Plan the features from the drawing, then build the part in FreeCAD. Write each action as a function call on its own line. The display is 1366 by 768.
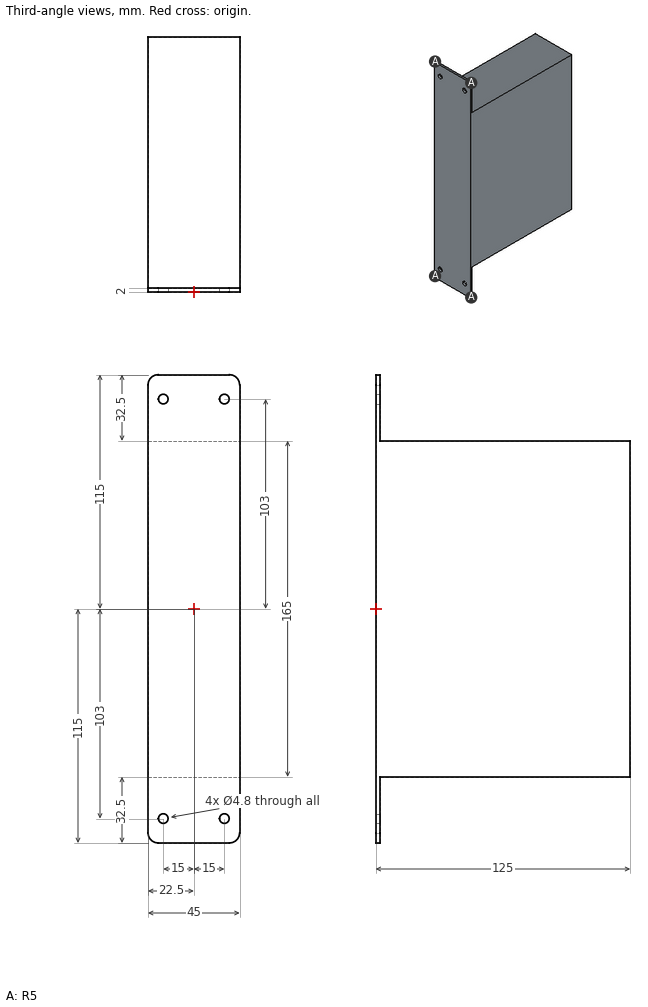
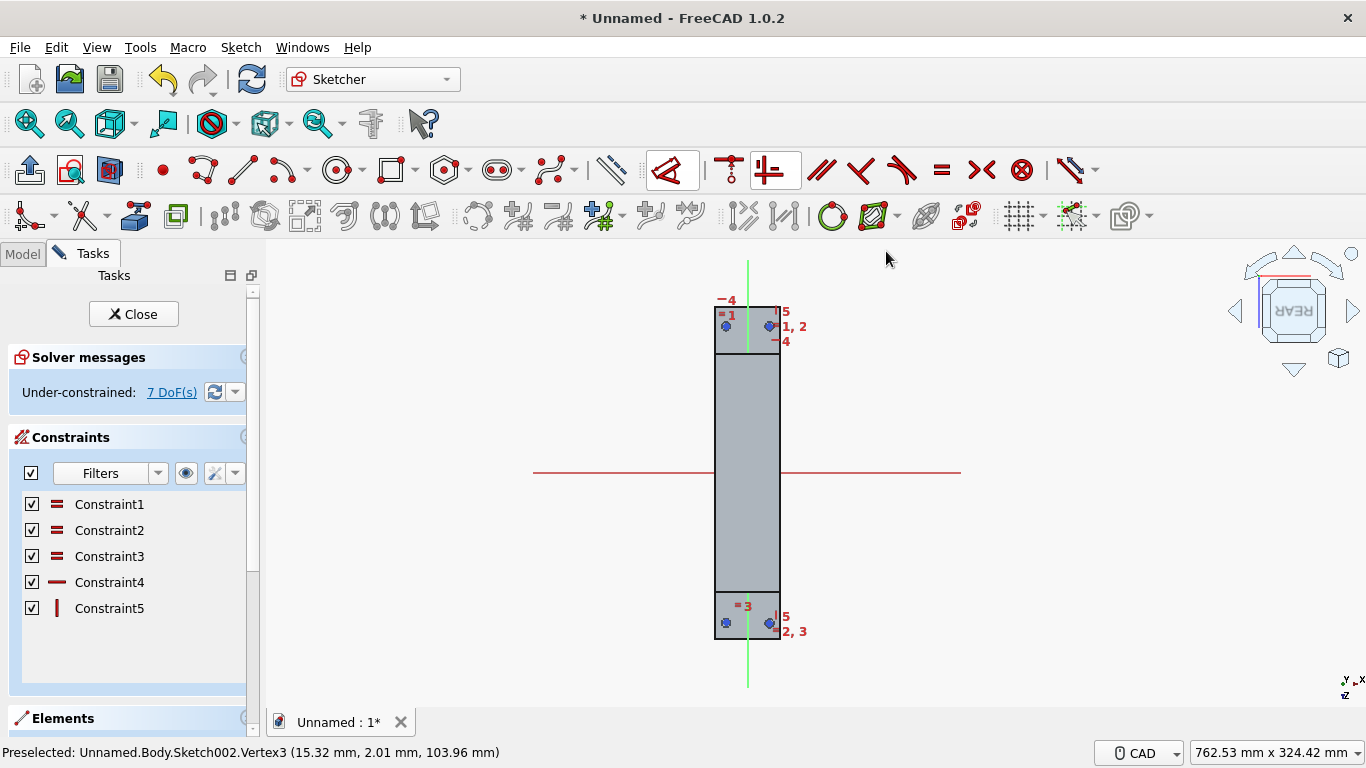
click(726, 326)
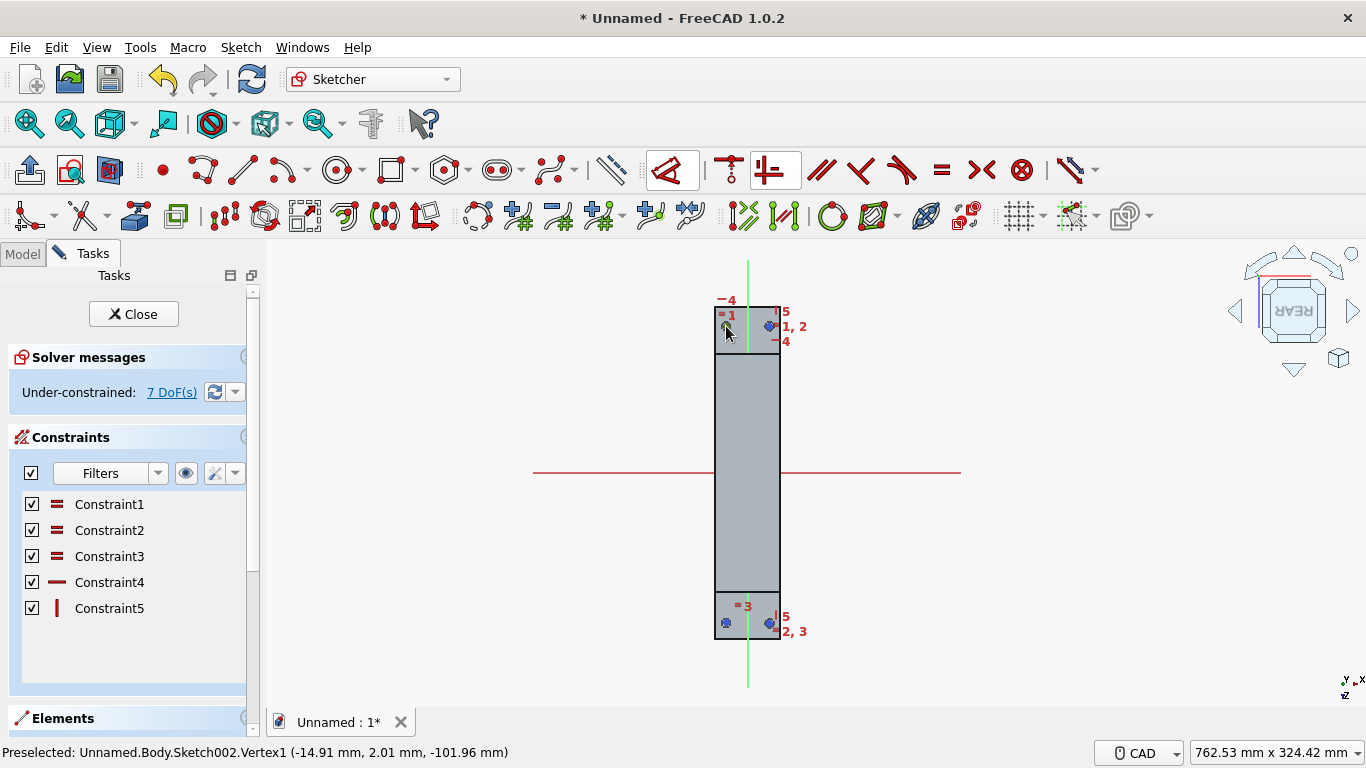
click(726, 623)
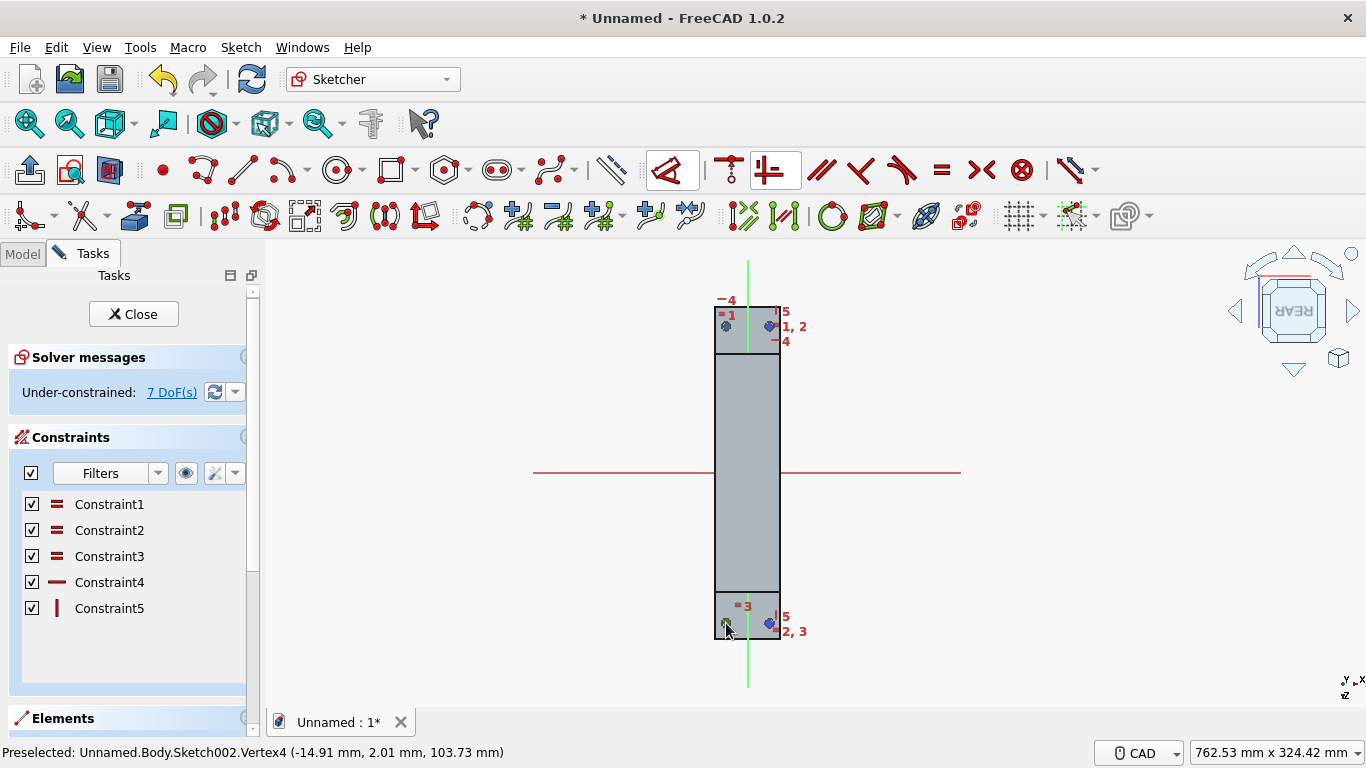
click(796, 170)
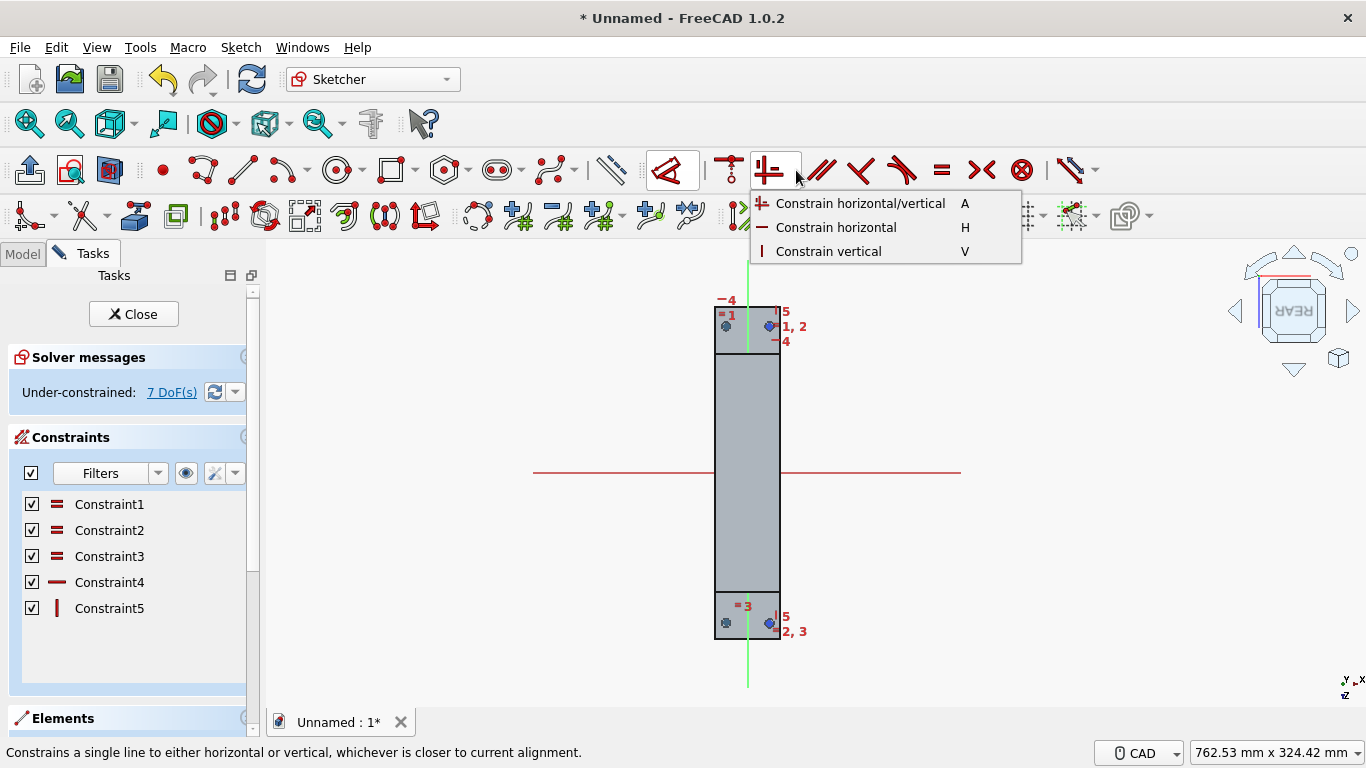
click(886, 251)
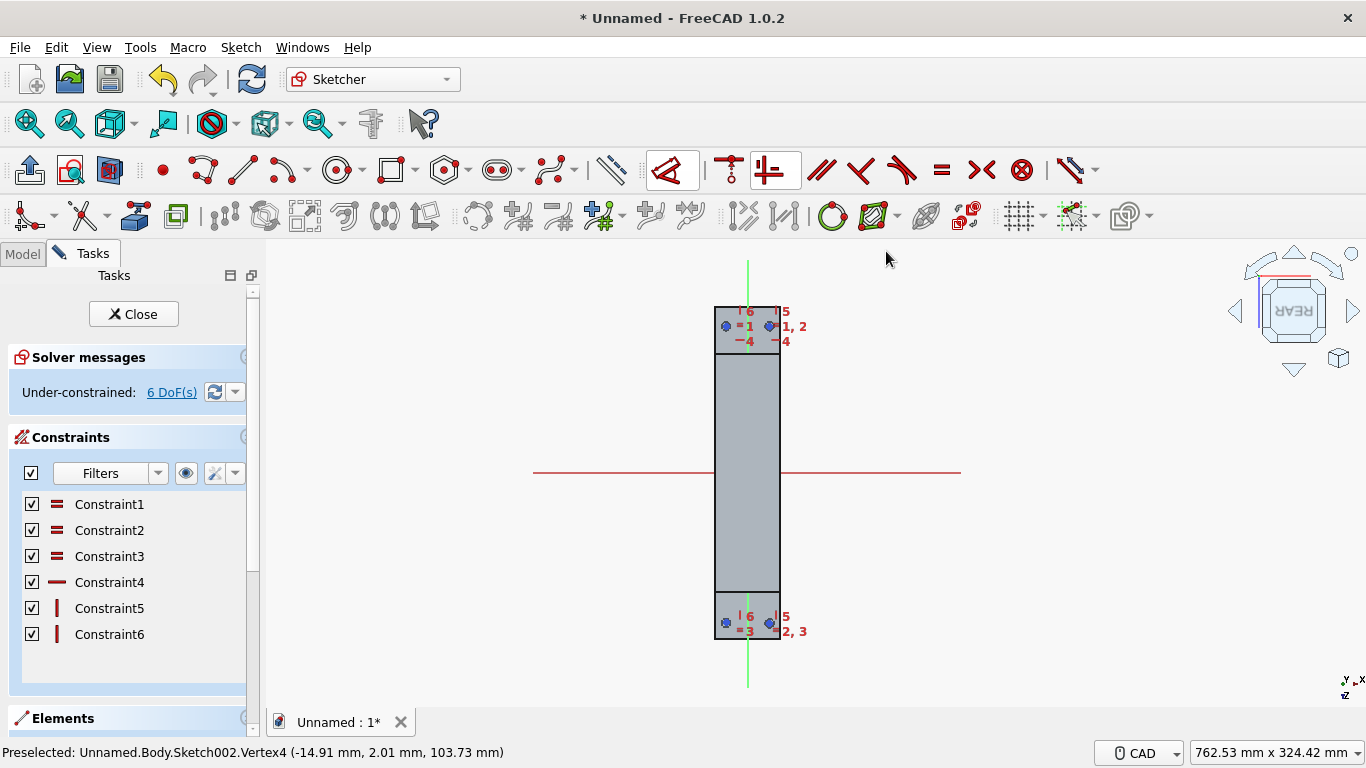
click(768, 625)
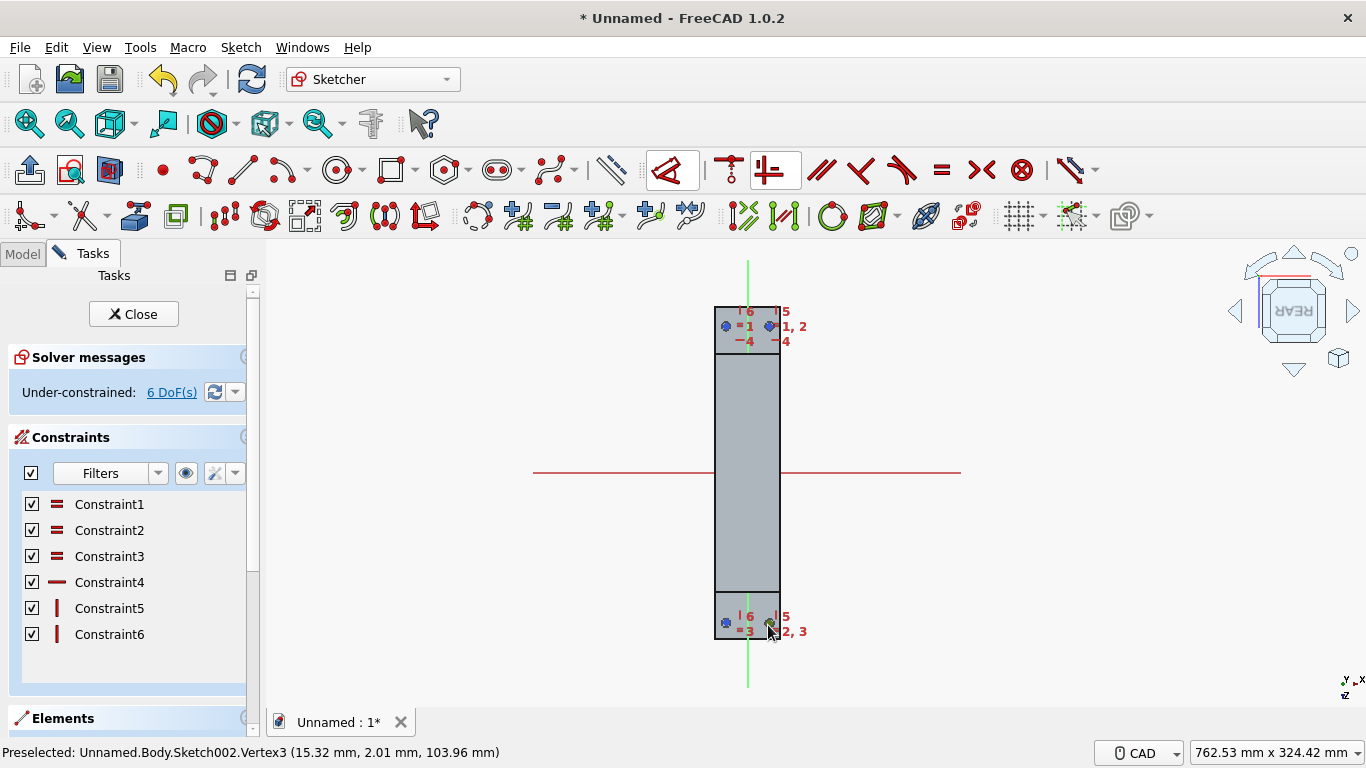
click(726, 623)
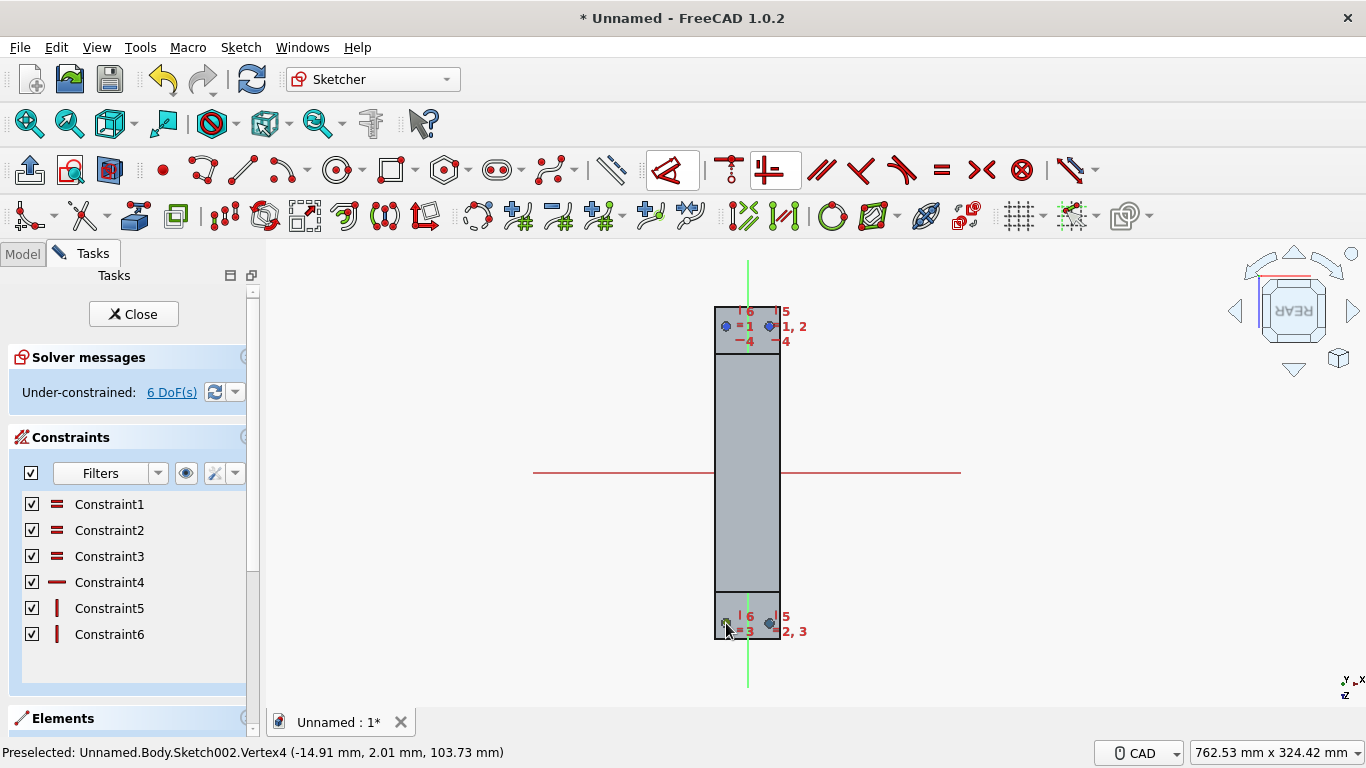
click(796, 170)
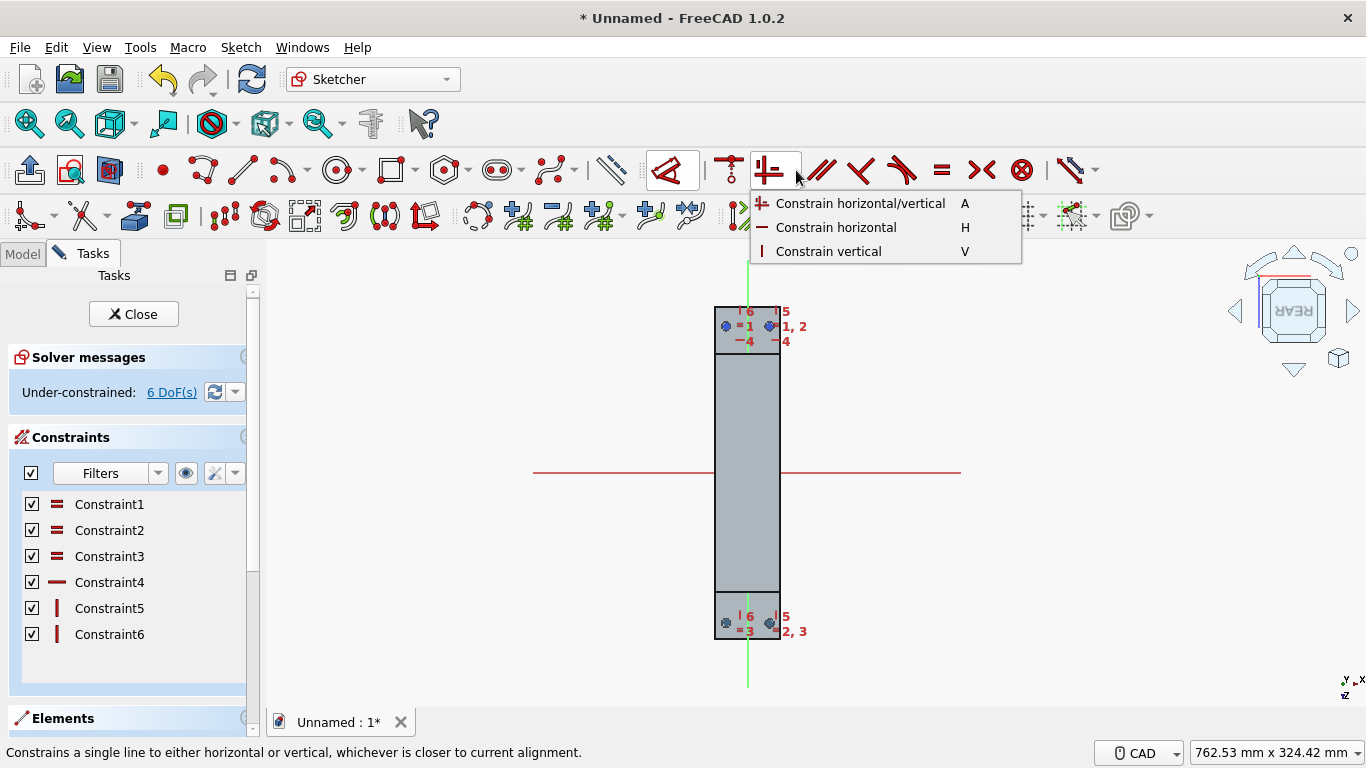
click(886, 227)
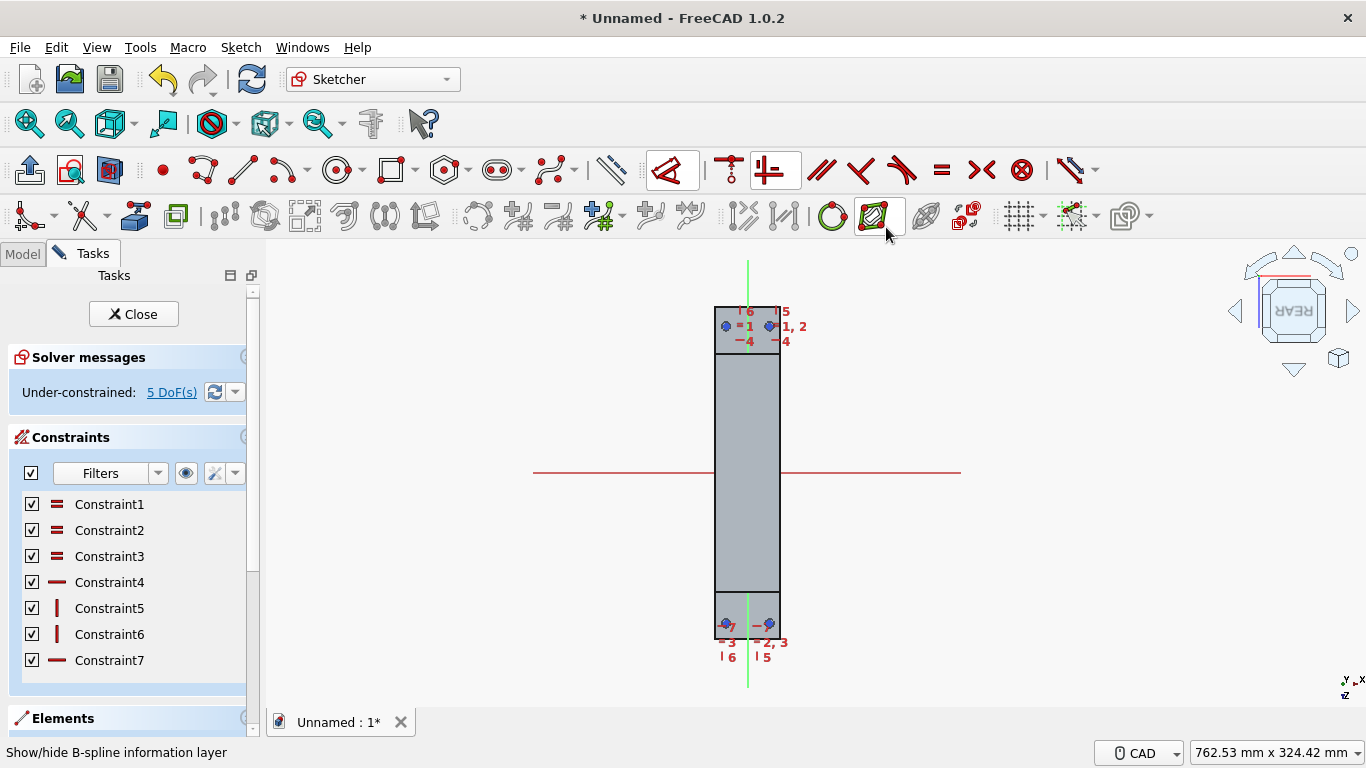
scroll(730, 326, up, 9)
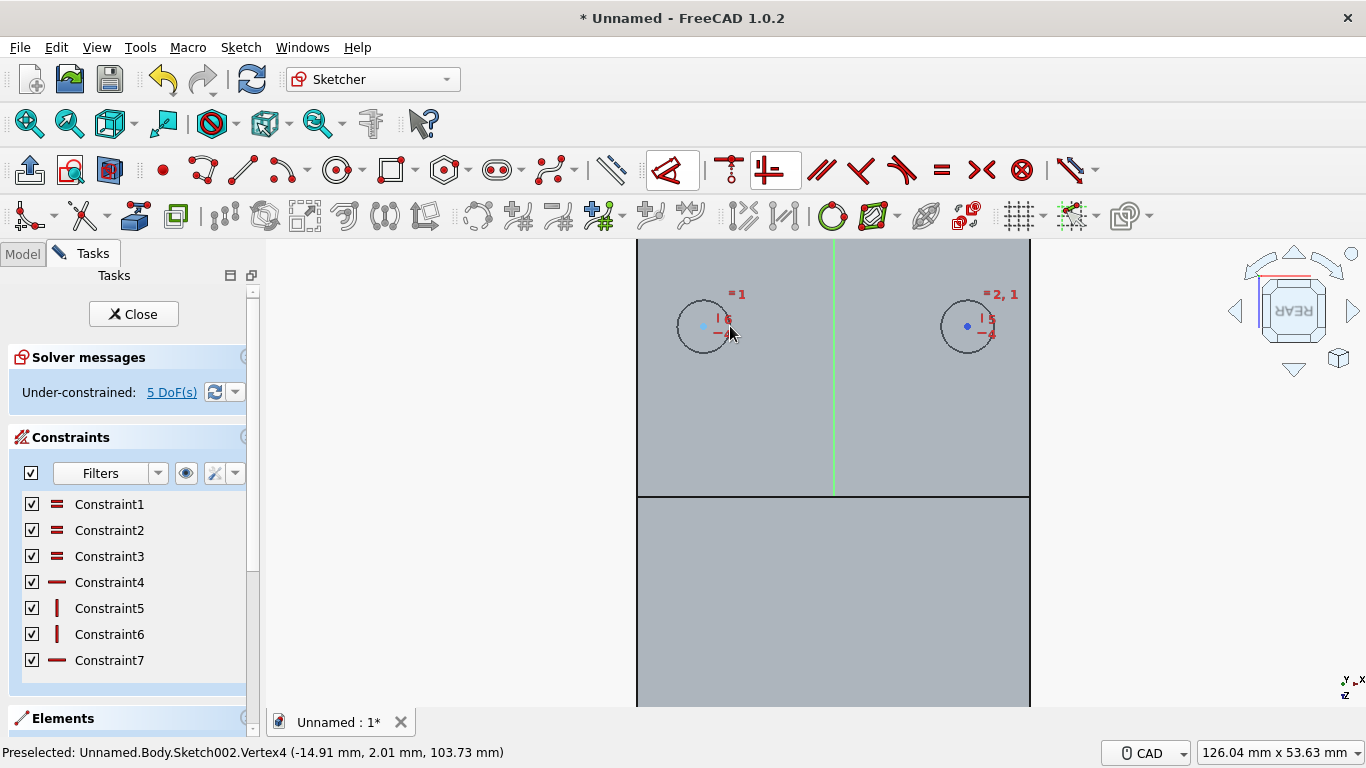
click(722, 308)